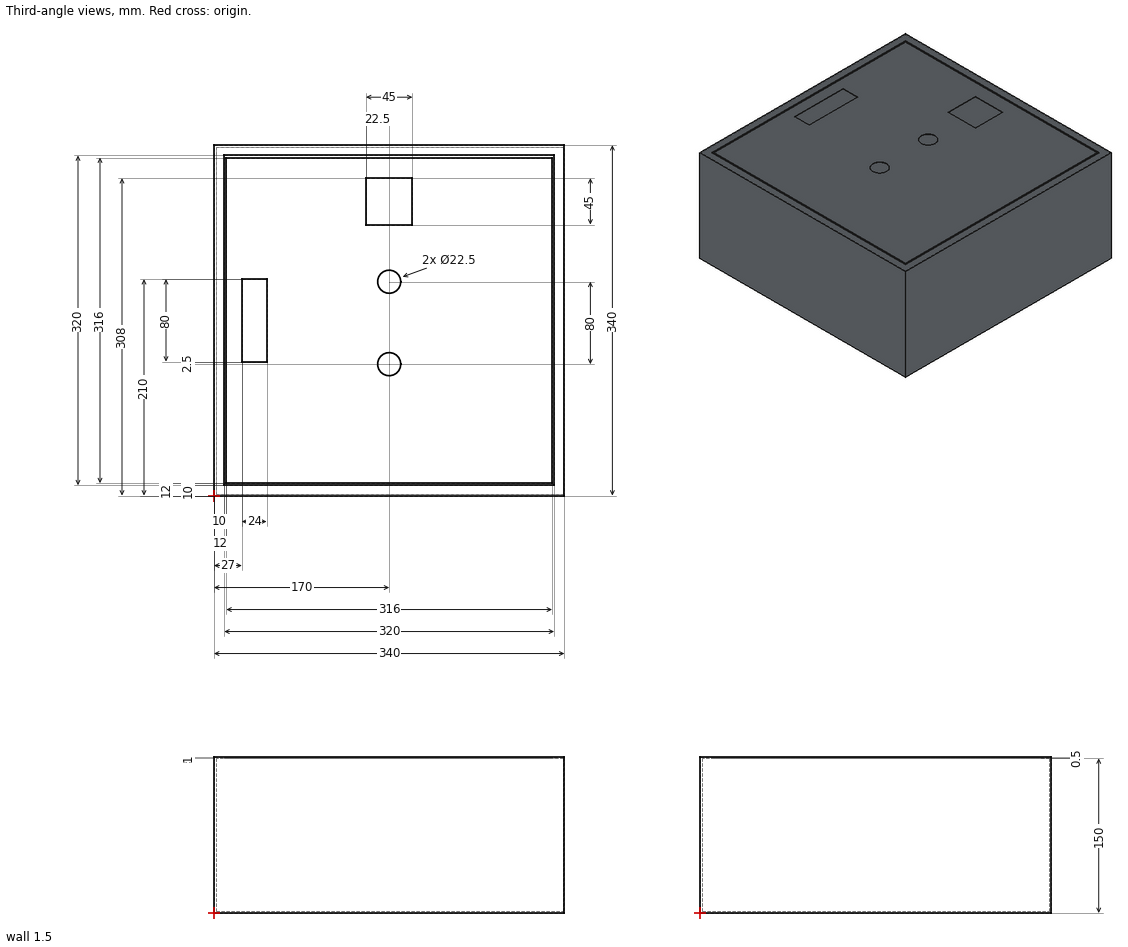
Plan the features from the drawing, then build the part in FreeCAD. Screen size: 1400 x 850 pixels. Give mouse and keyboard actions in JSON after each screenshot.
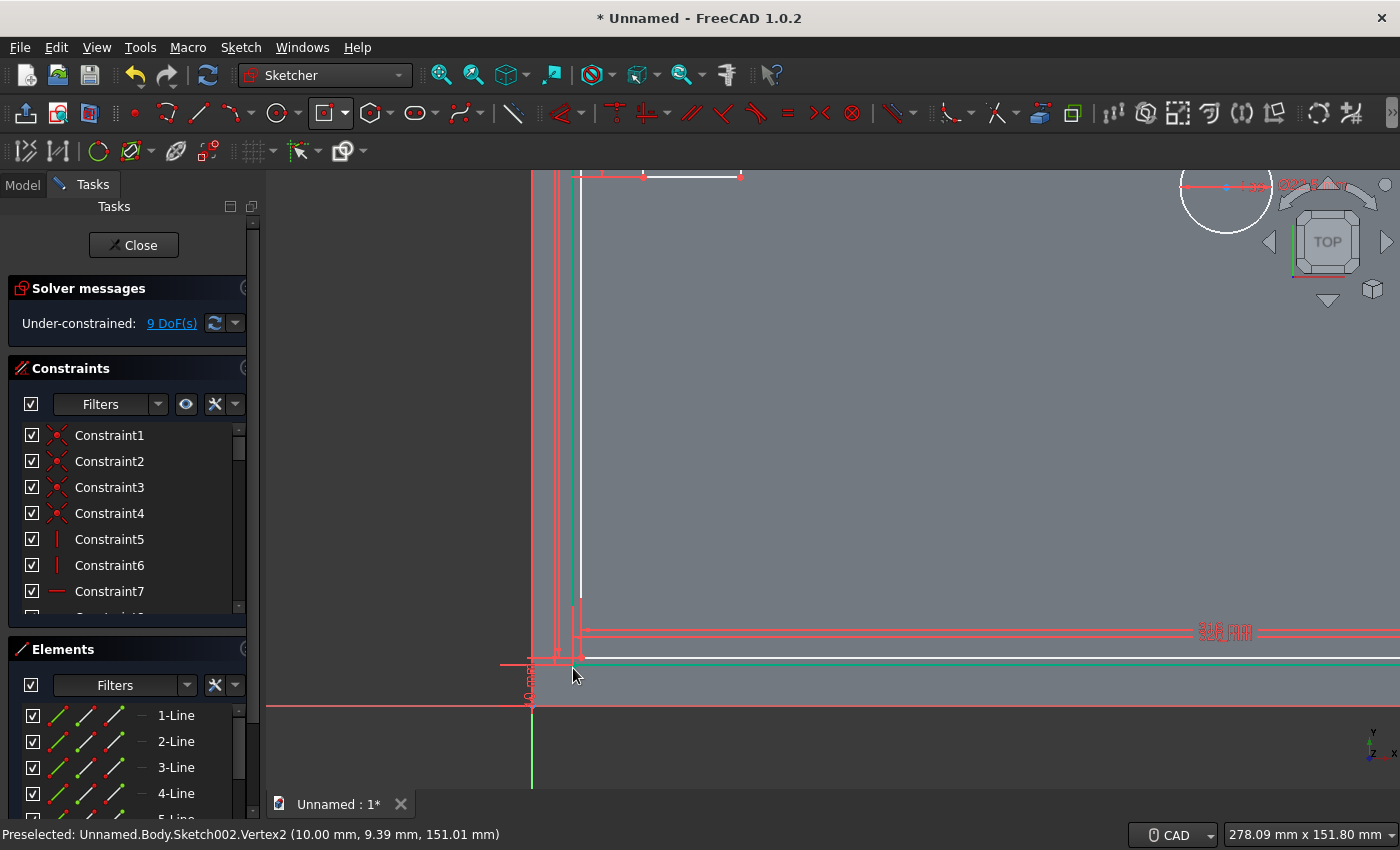
{"action": "scroll", "coordinate": [575, 672], "scroll_direction": "down", "scroll_amount": 6}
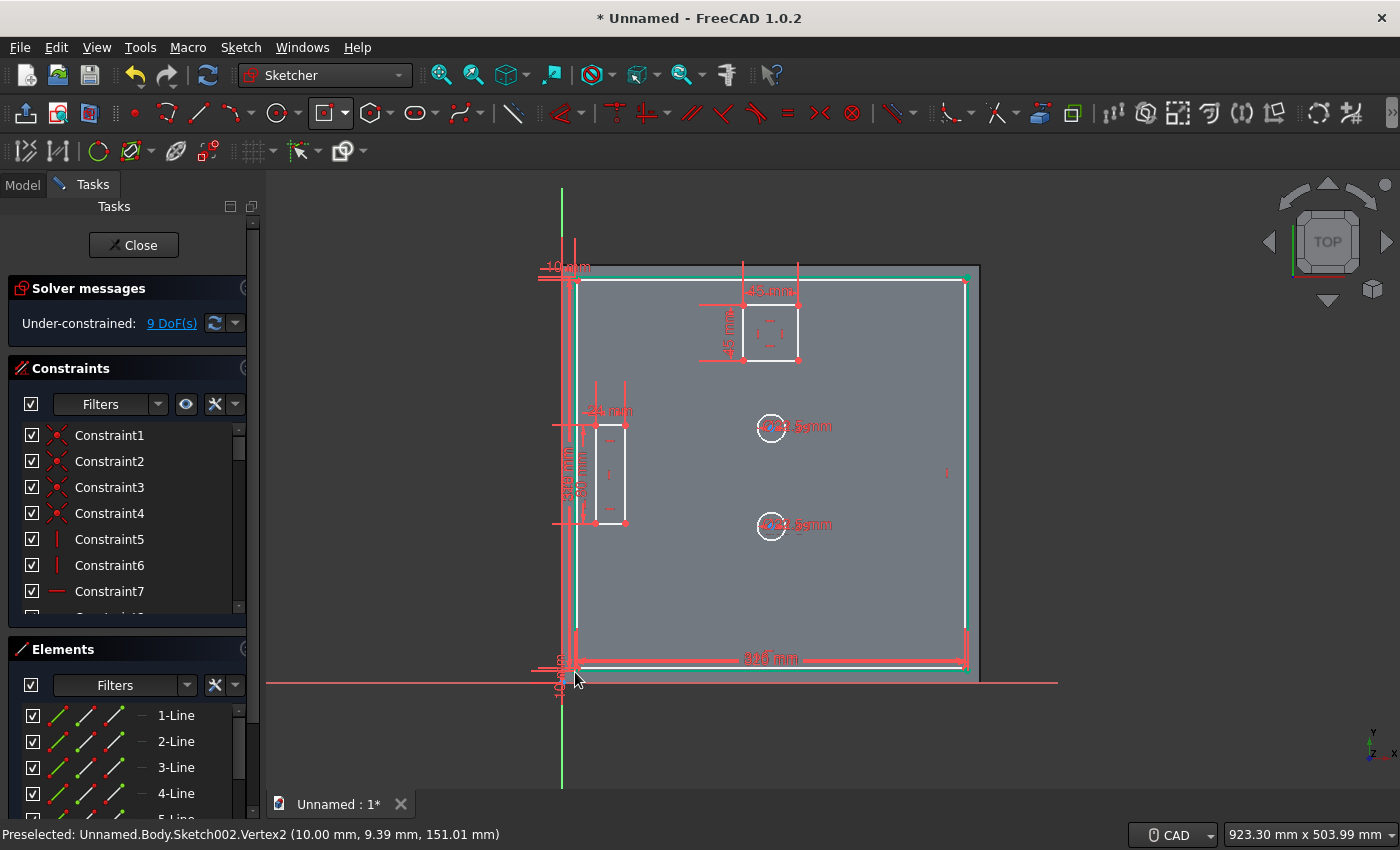
{"action": "left_click", "coordinate": [596, 425]}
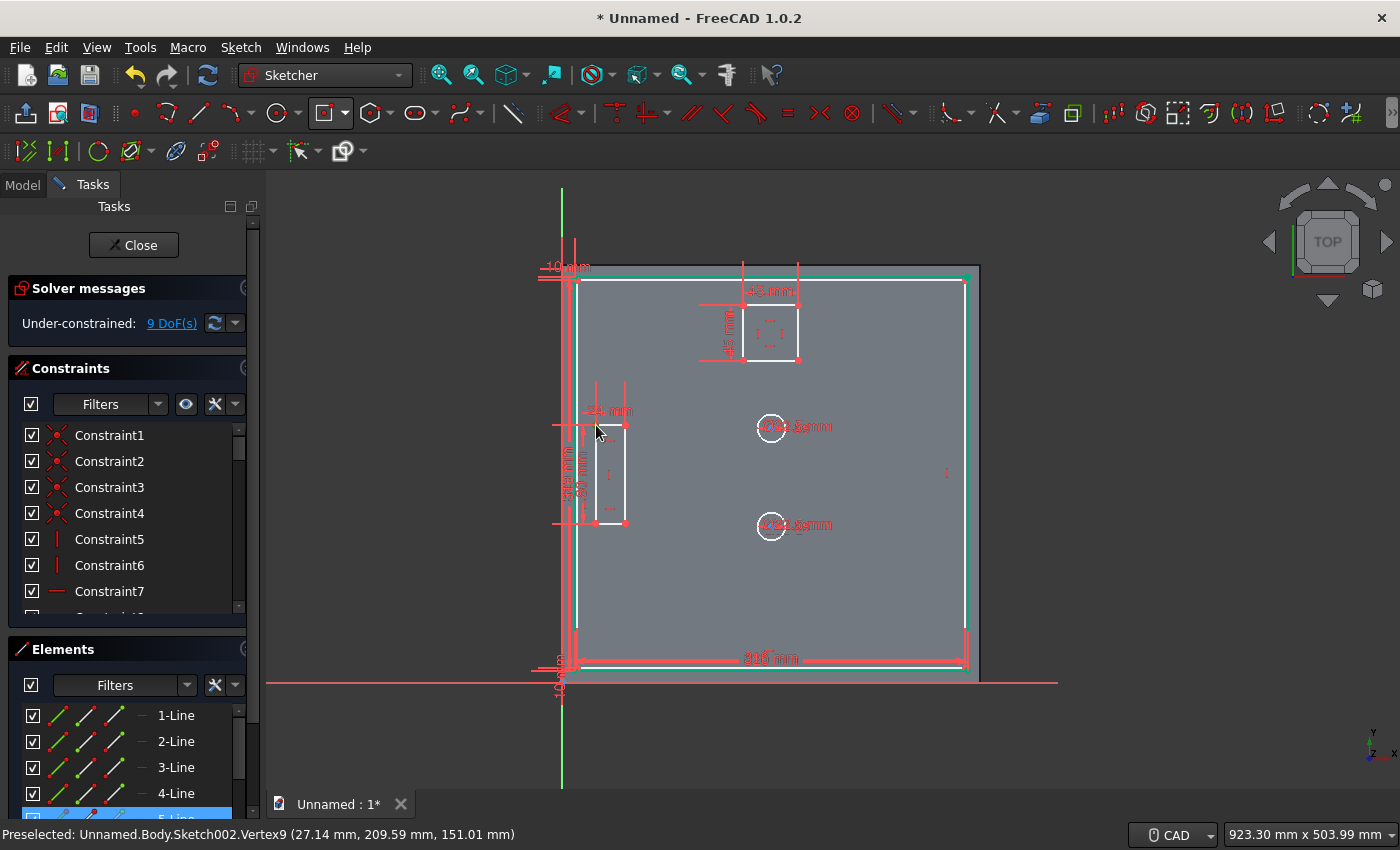
{"action": "key", "text": "l"}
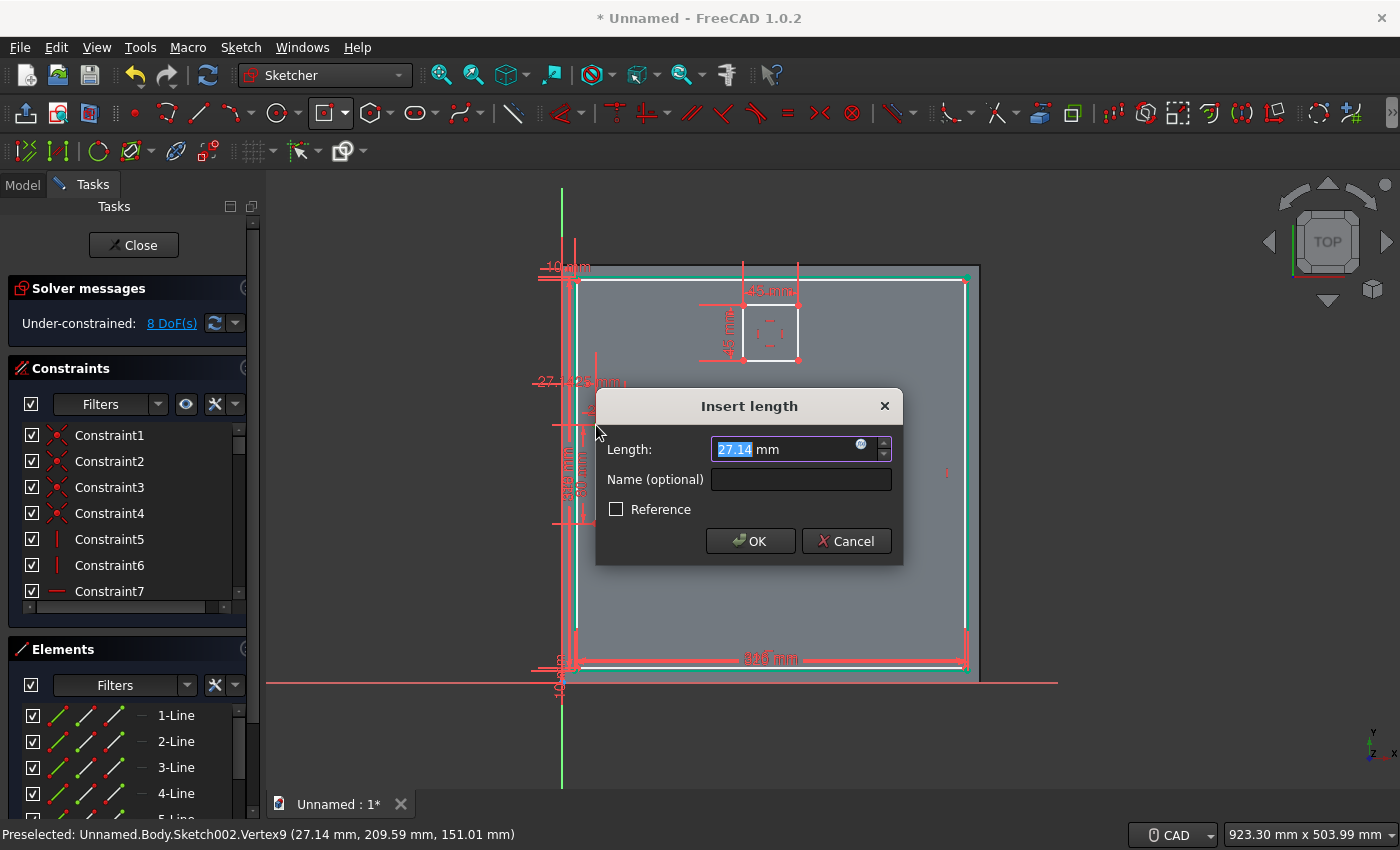
{"action": "type", "text": "27"}
{"action": "key", "text": "Return"}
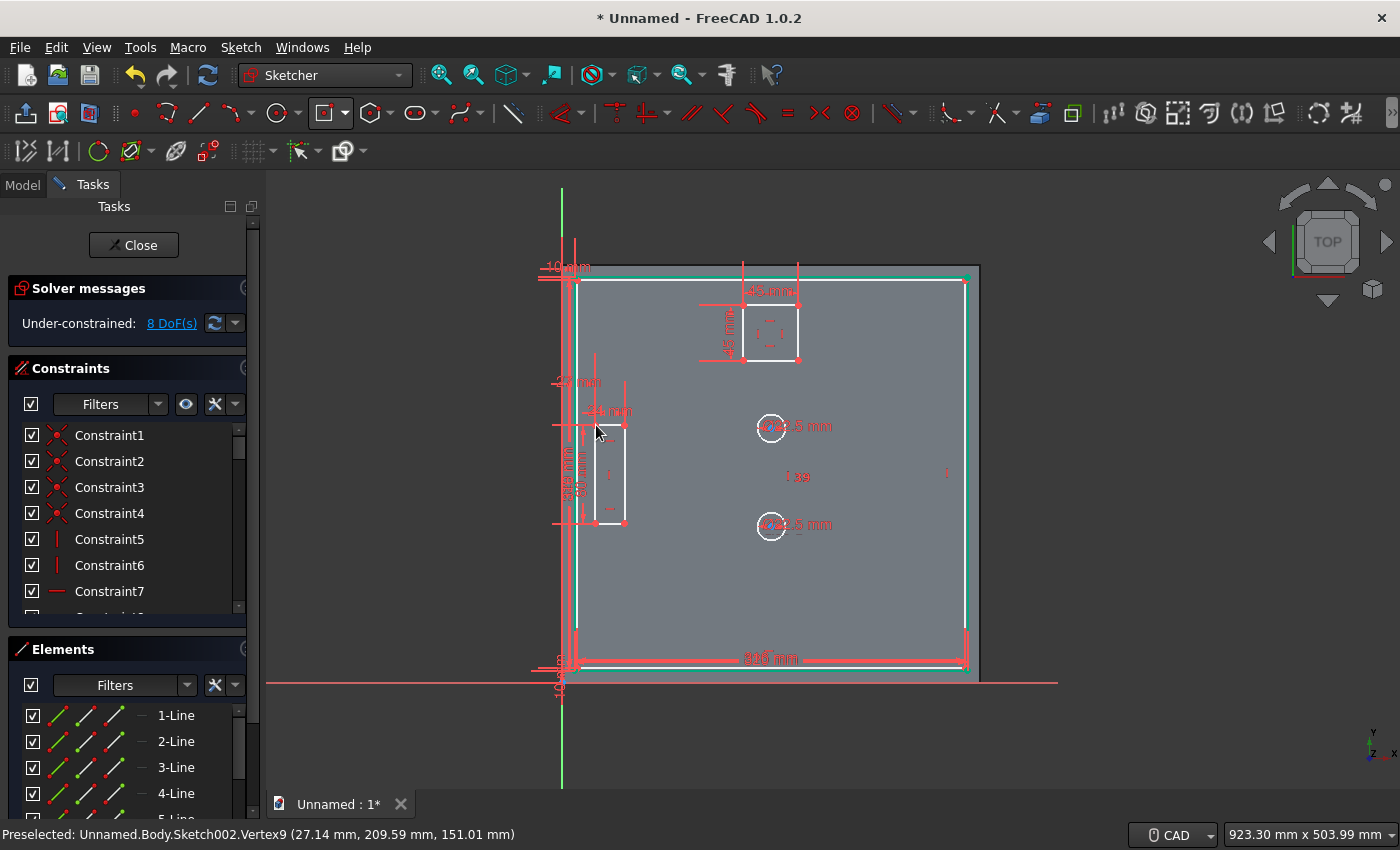
{"action": "scroll", "coordinate": [577, 280], "scroll_direction": "up", "scroll_amount": 7}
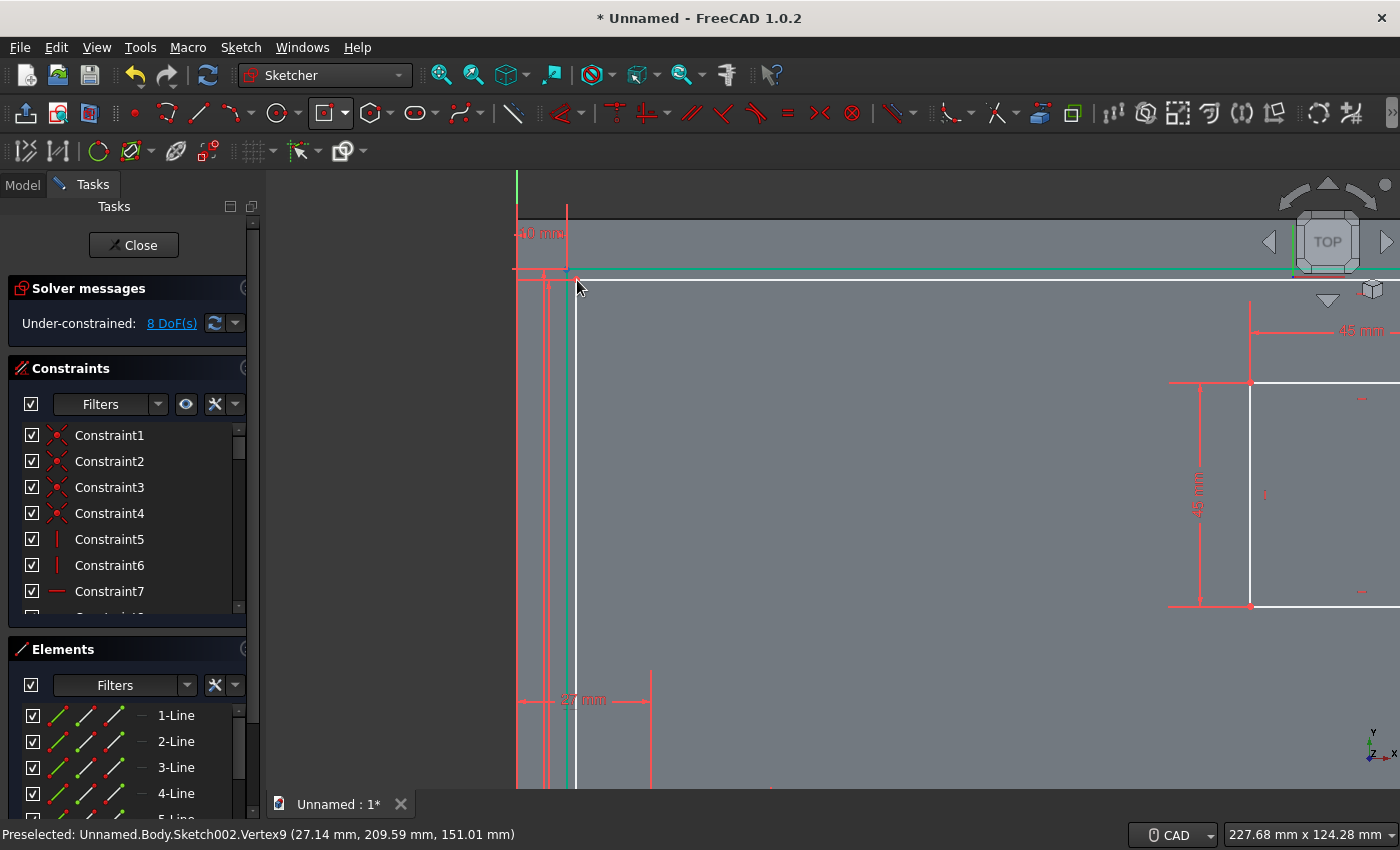
{"action": "left_click", "coordinate": [576, 280]}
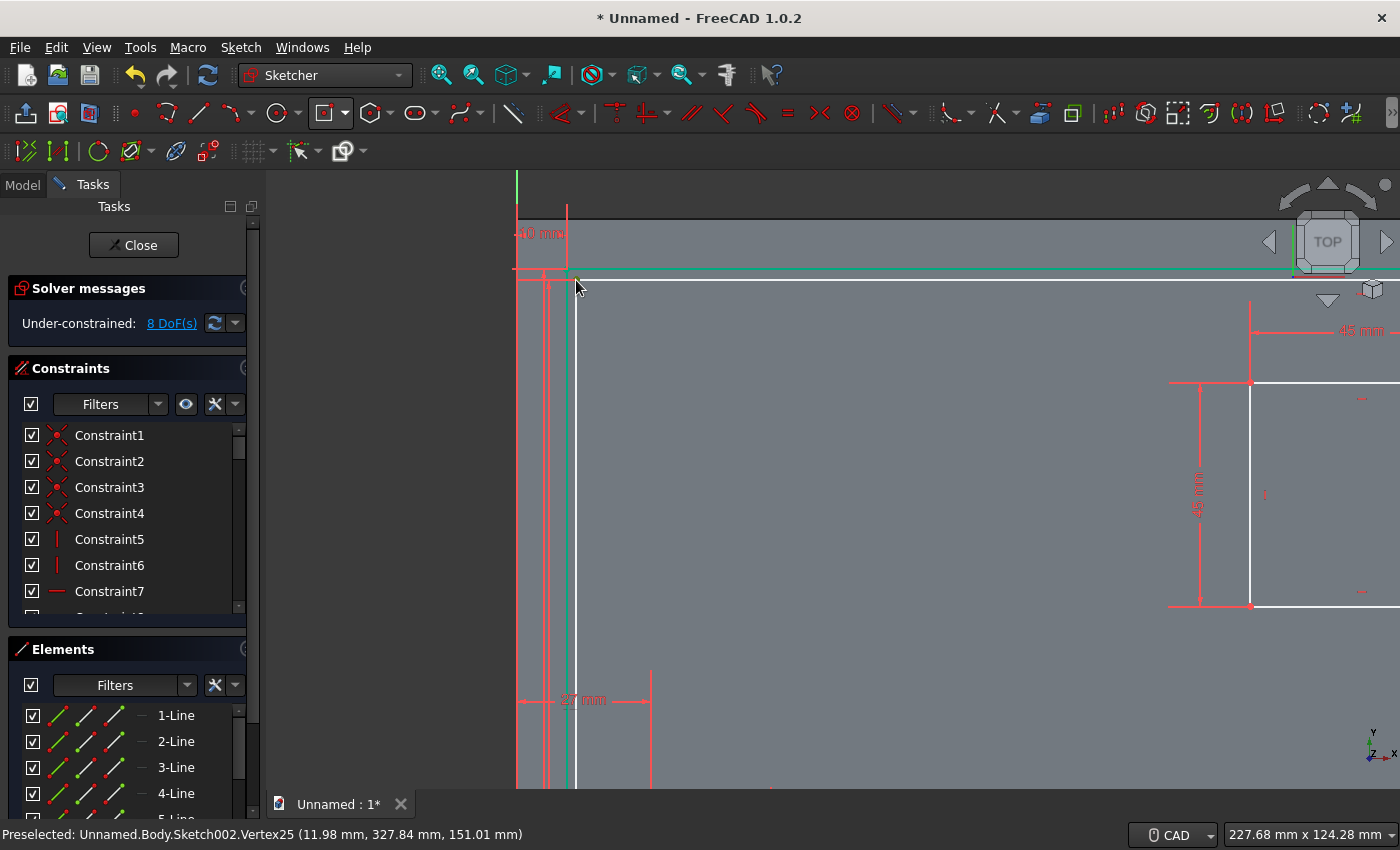
{"action": "key", "text": "l"}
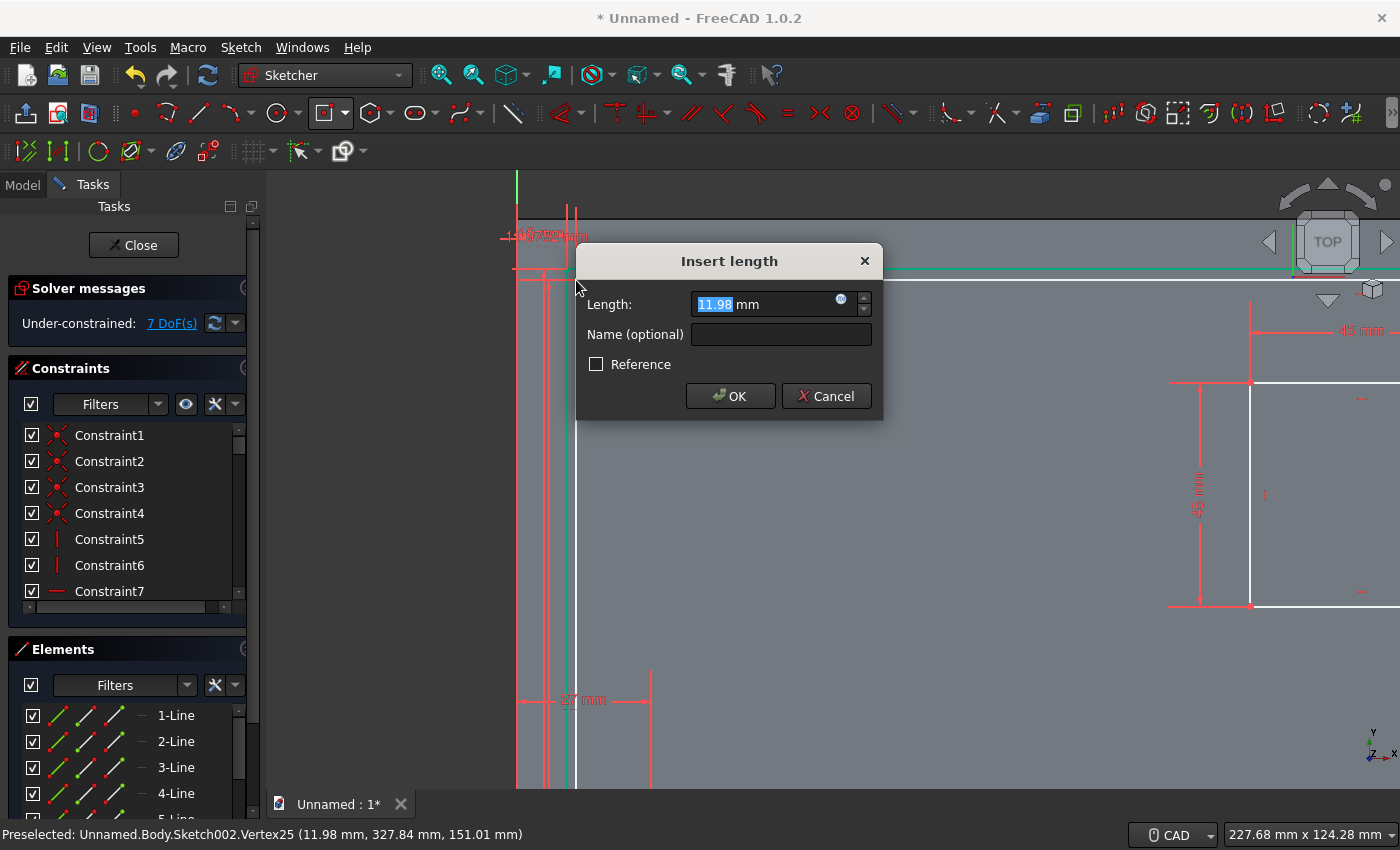
{"action": "type", "text": "12"}
{"action": "key", "text": "Return"}